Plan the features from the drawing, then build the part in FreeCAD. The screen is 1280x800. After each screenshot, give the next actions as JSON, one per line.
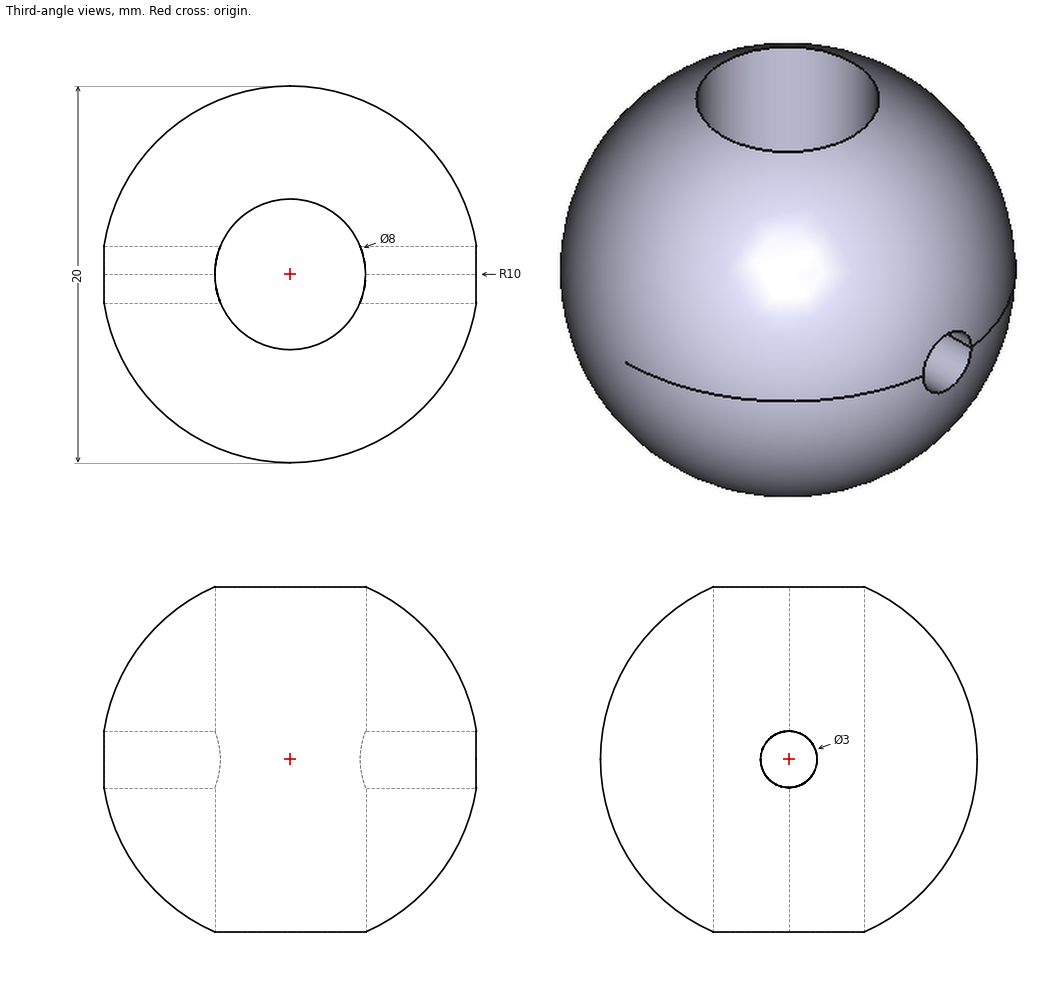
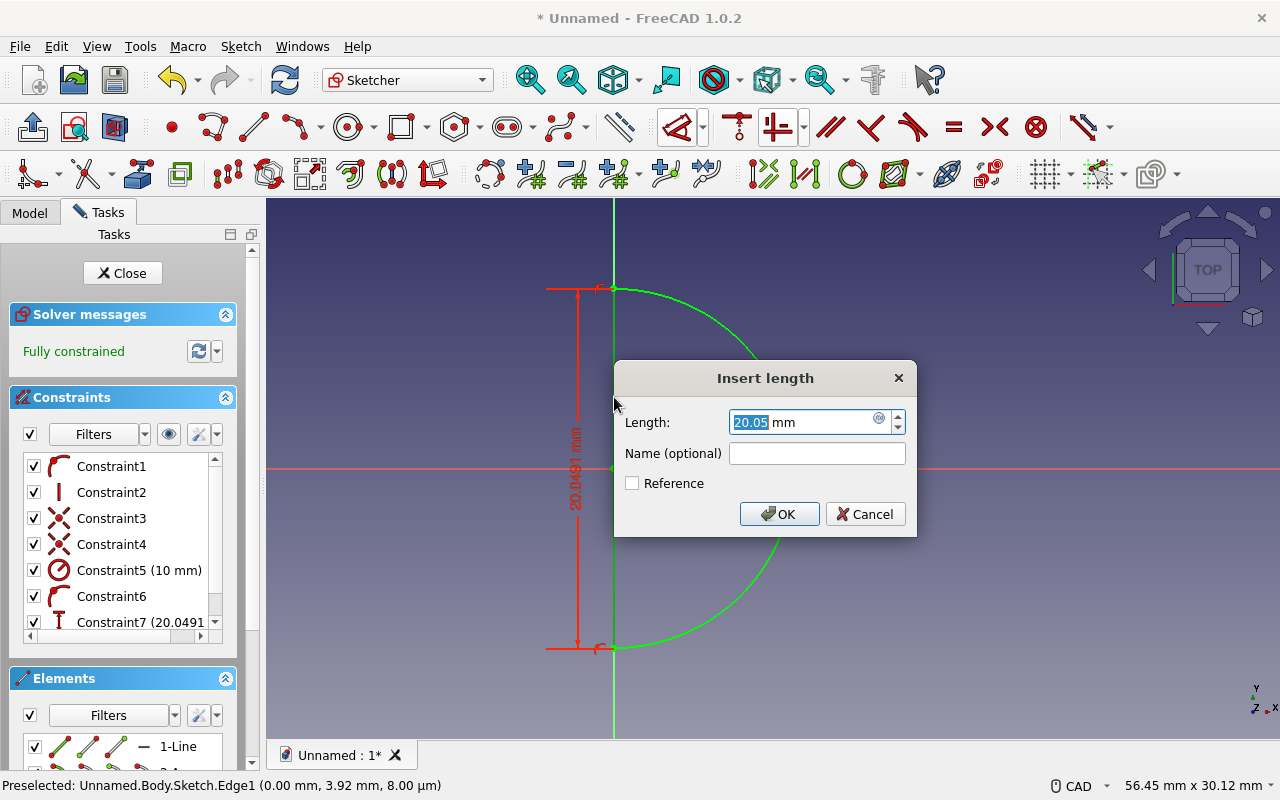
{"action": "type", "text": "20"}
{"action": "key", "text": "Return"}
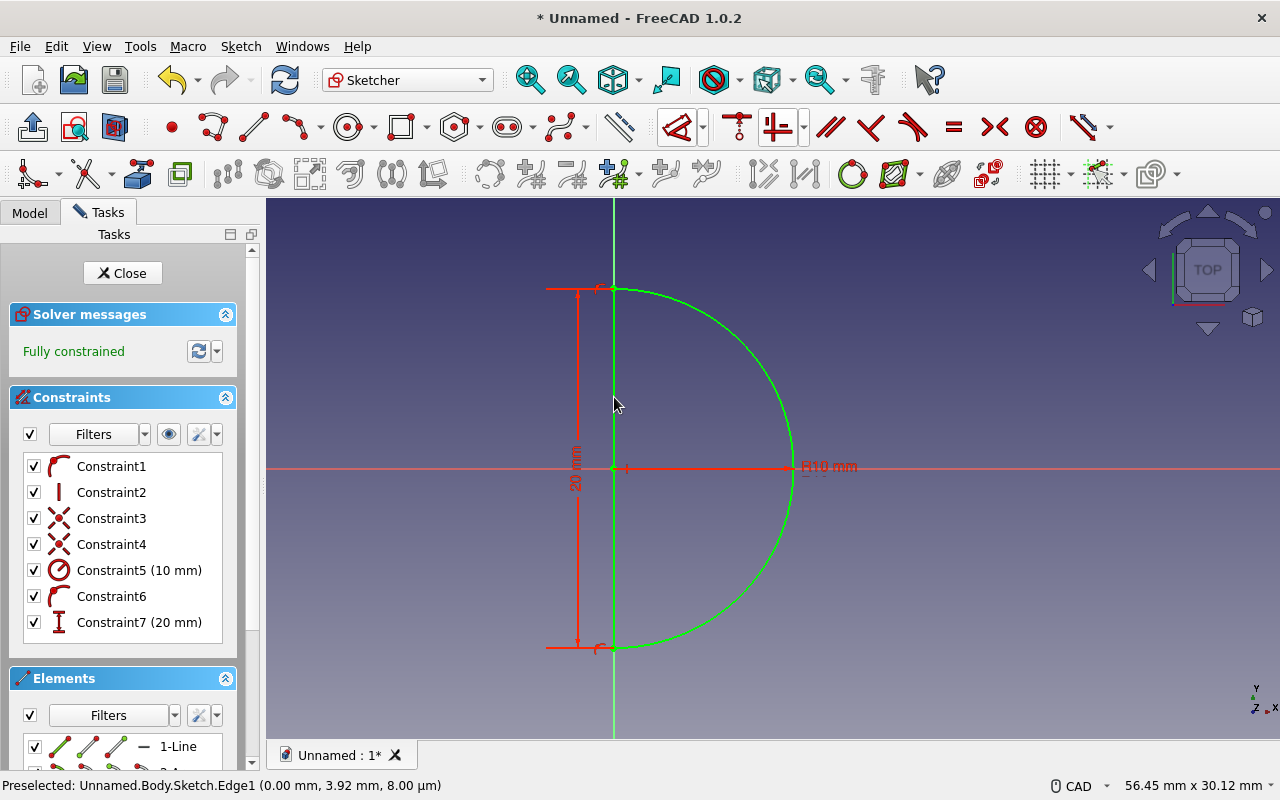
{"action": "left_click", "coordinate": [123, 273]}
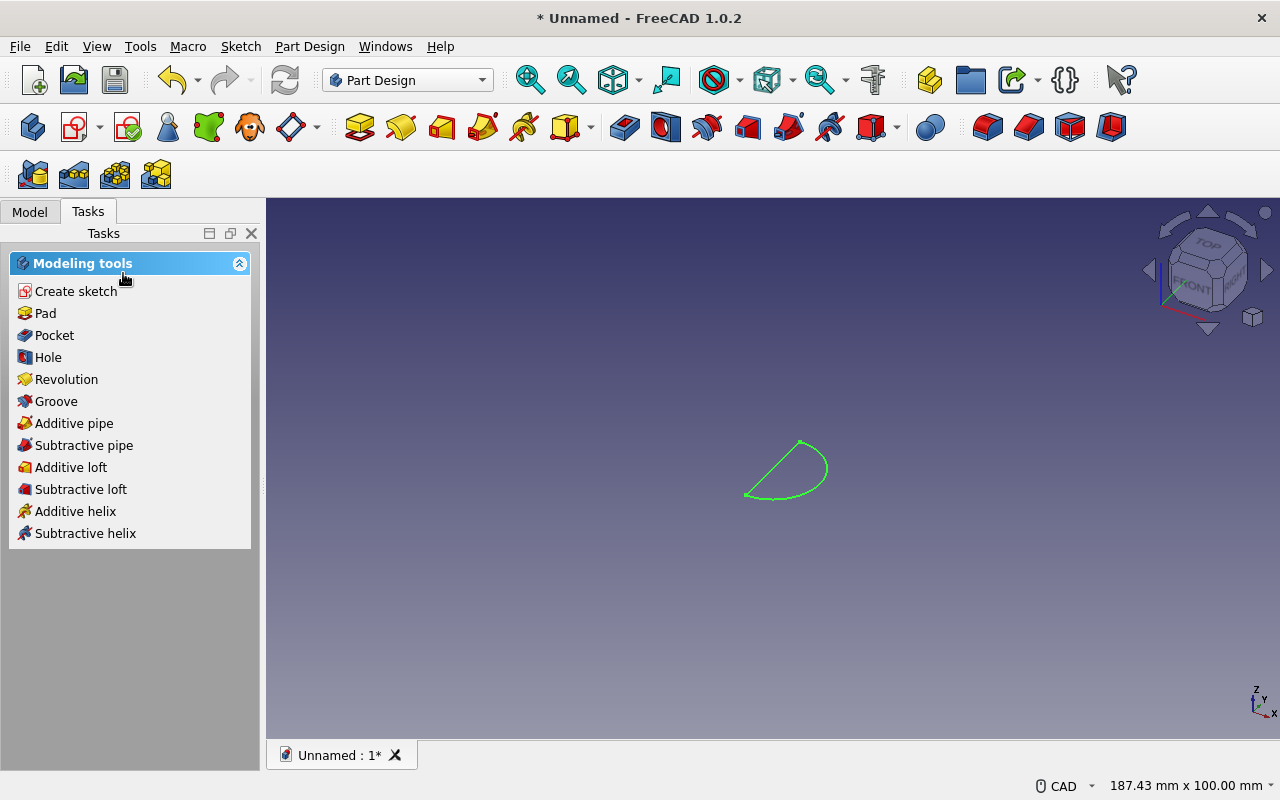
{"action": "left_click", "coordinate": [401, 128]}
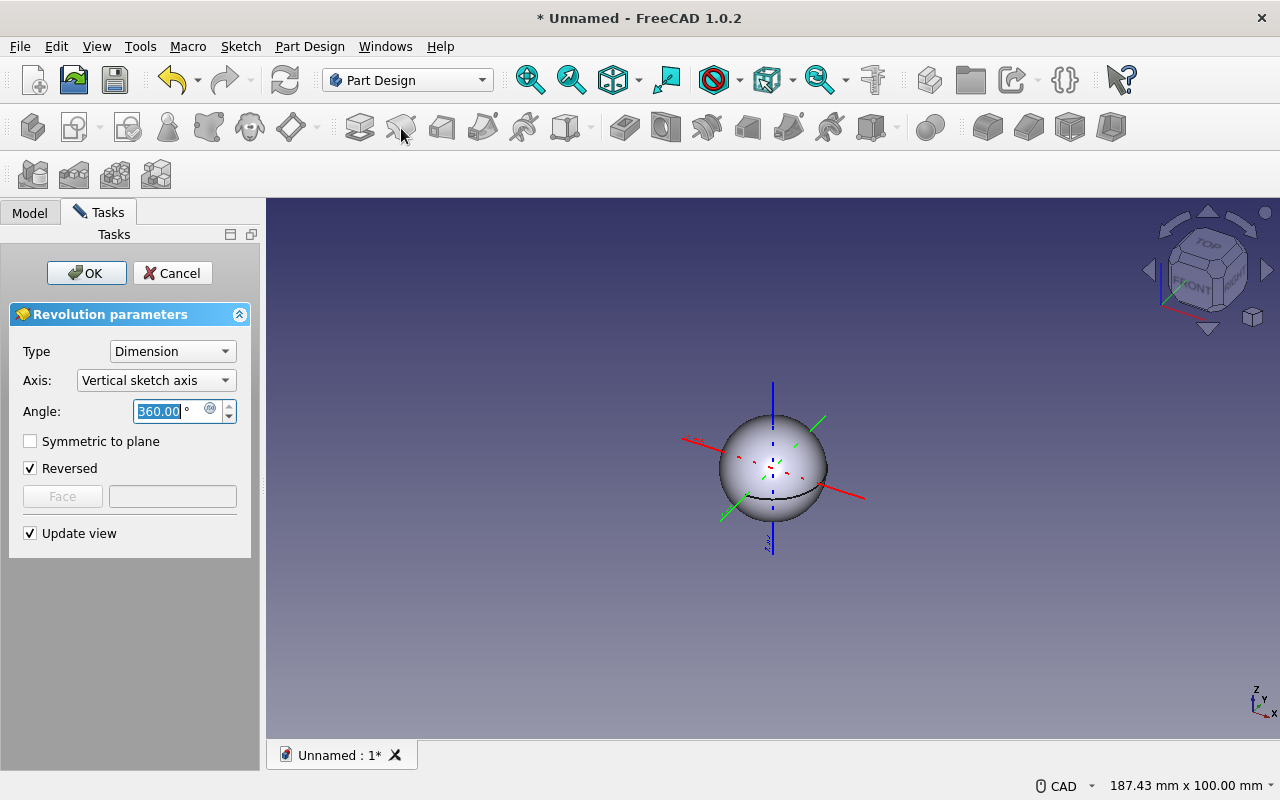
{"action": "left_click", "coordinate": [87, 273]}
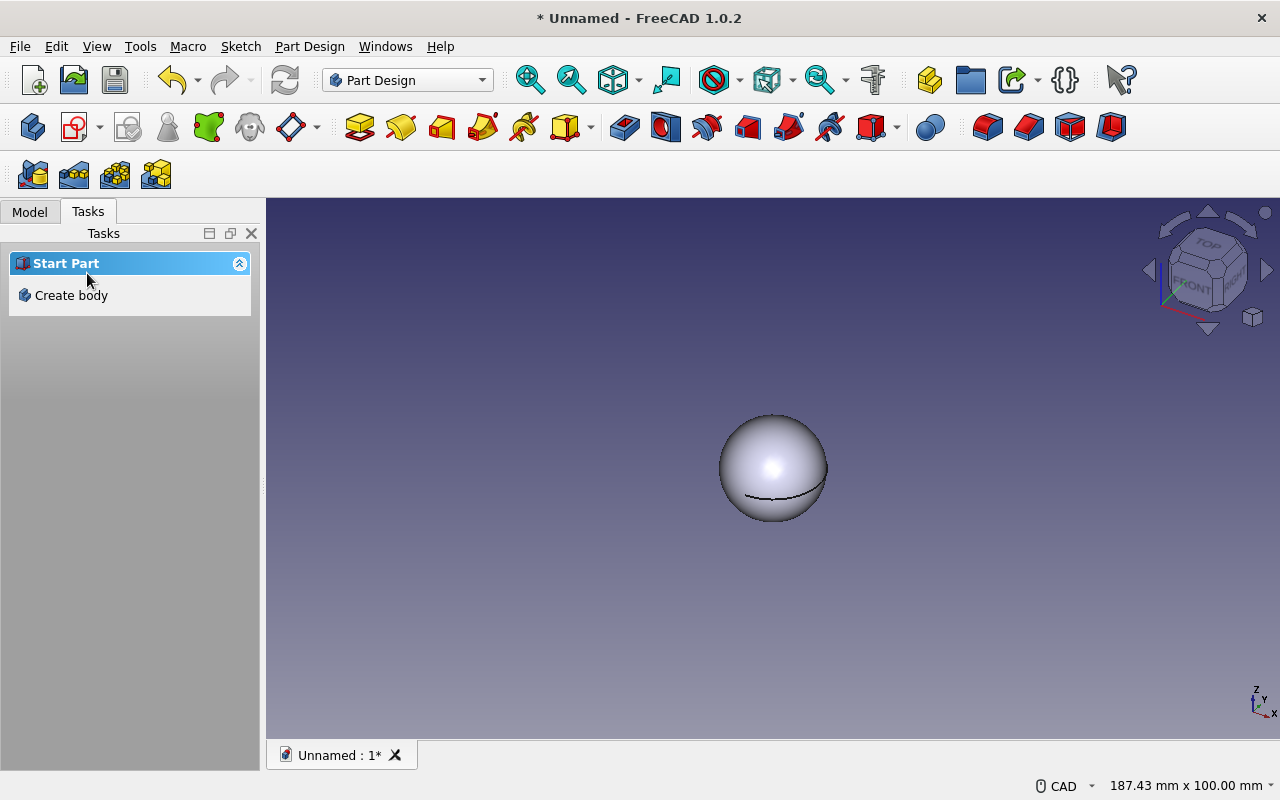
{"action": "left_click", "coordinate": [531, 80]}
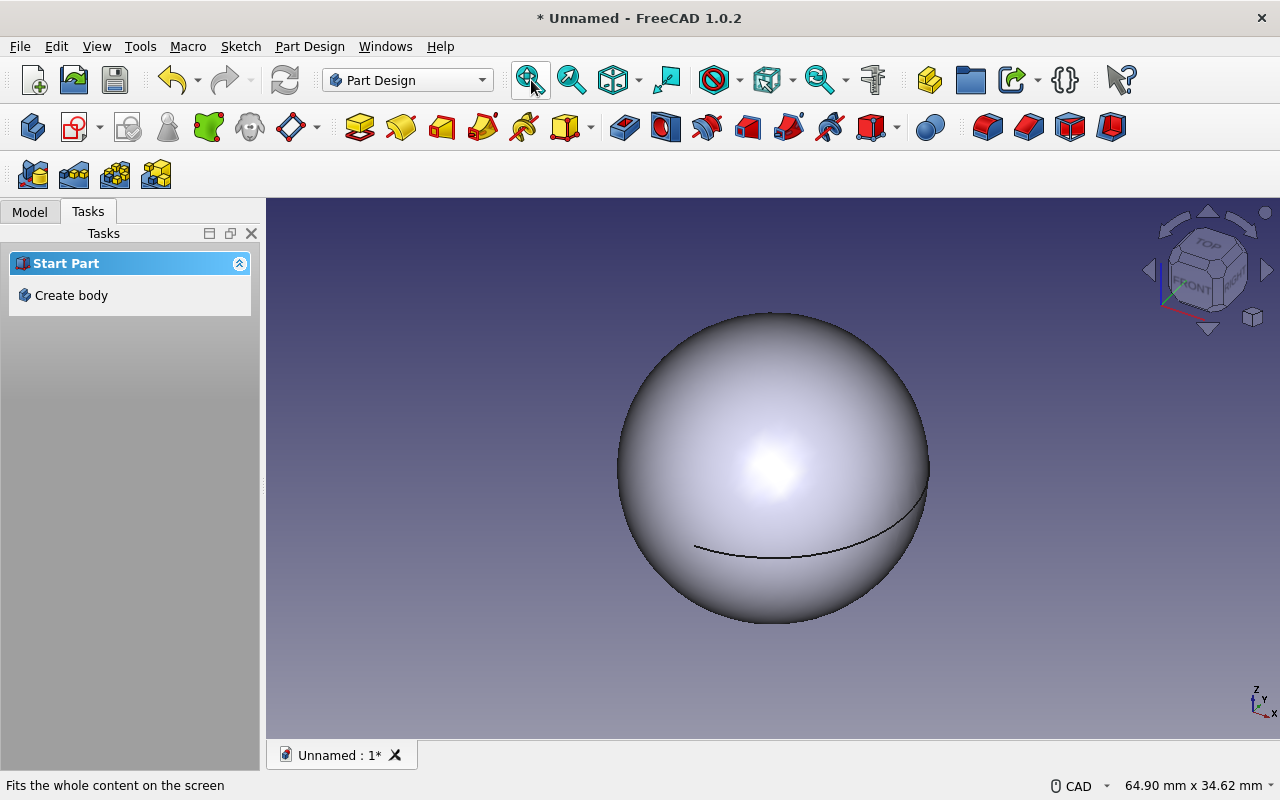
{"action": "left_click", "coordinate": [74, 128]}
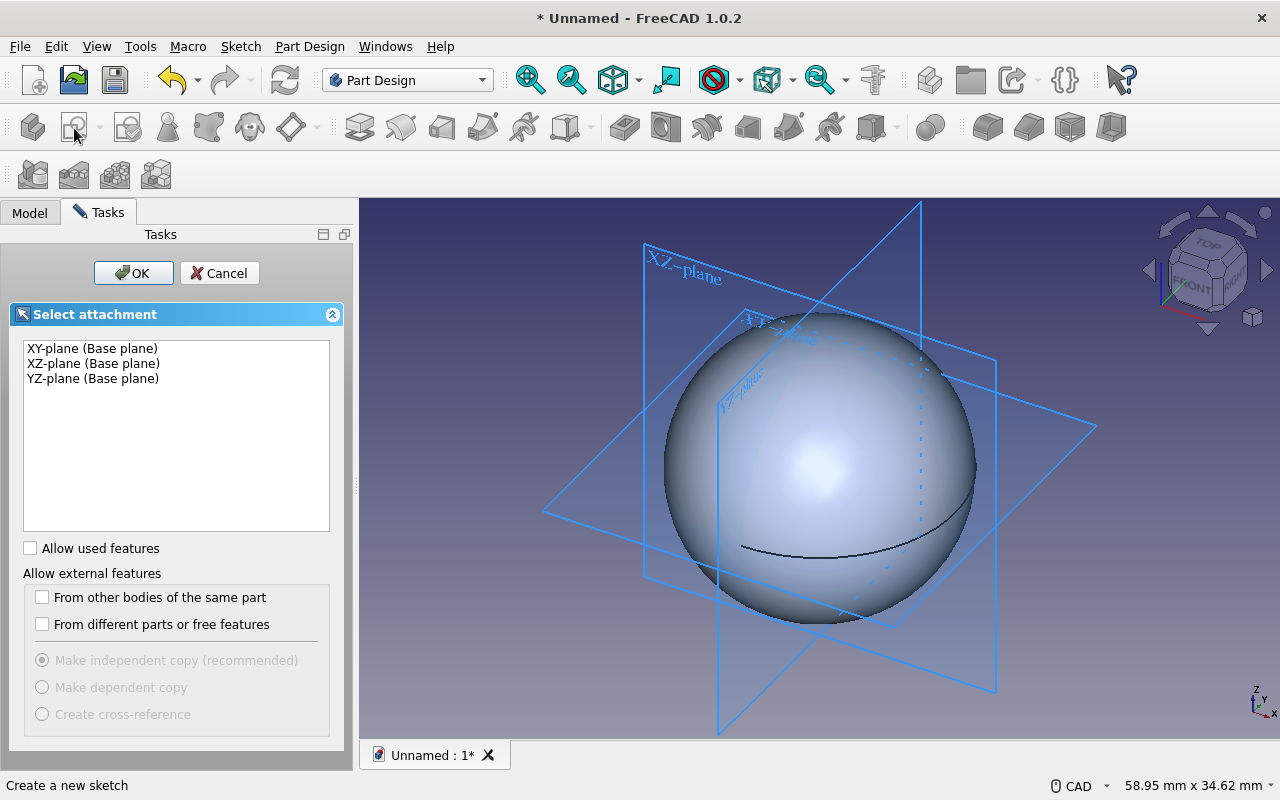
{"action": "left_click", "coordinate": [84, 348]}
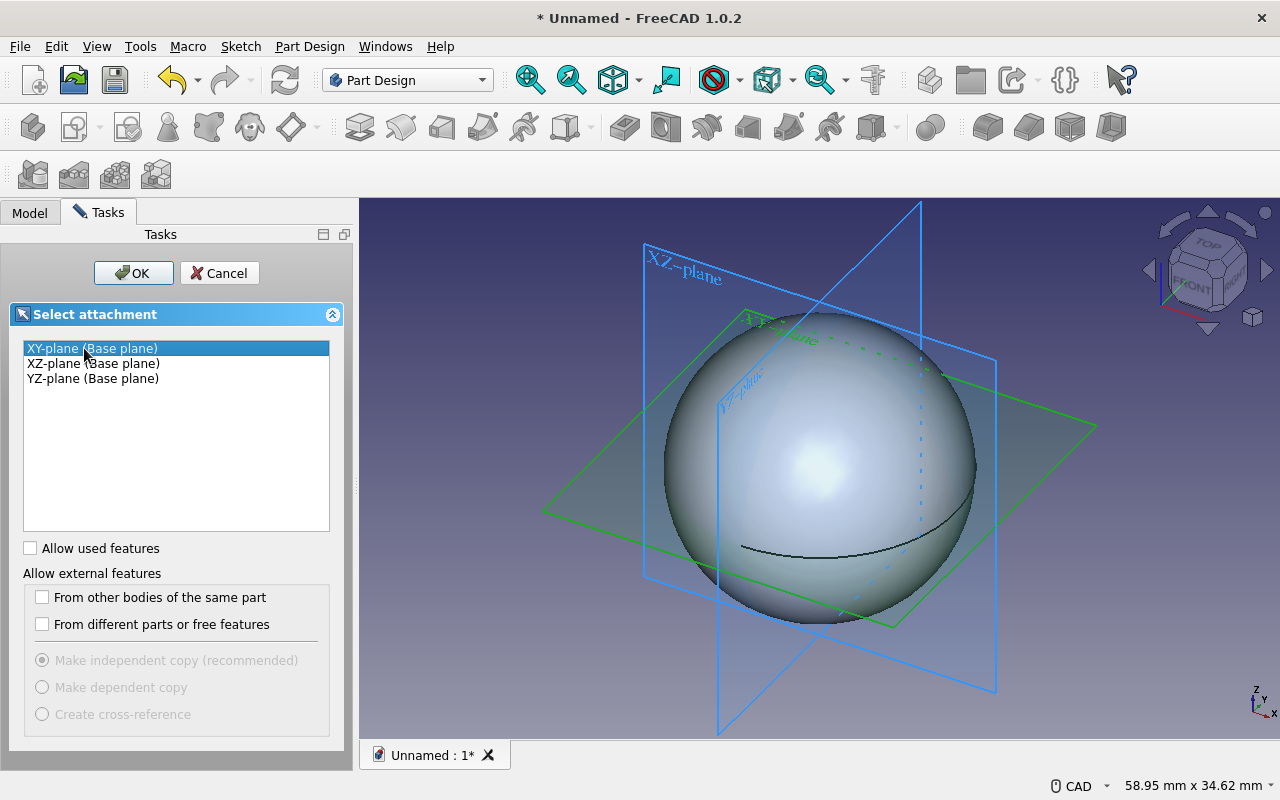
{"action": "left_click", "coordinate": [134, 273]}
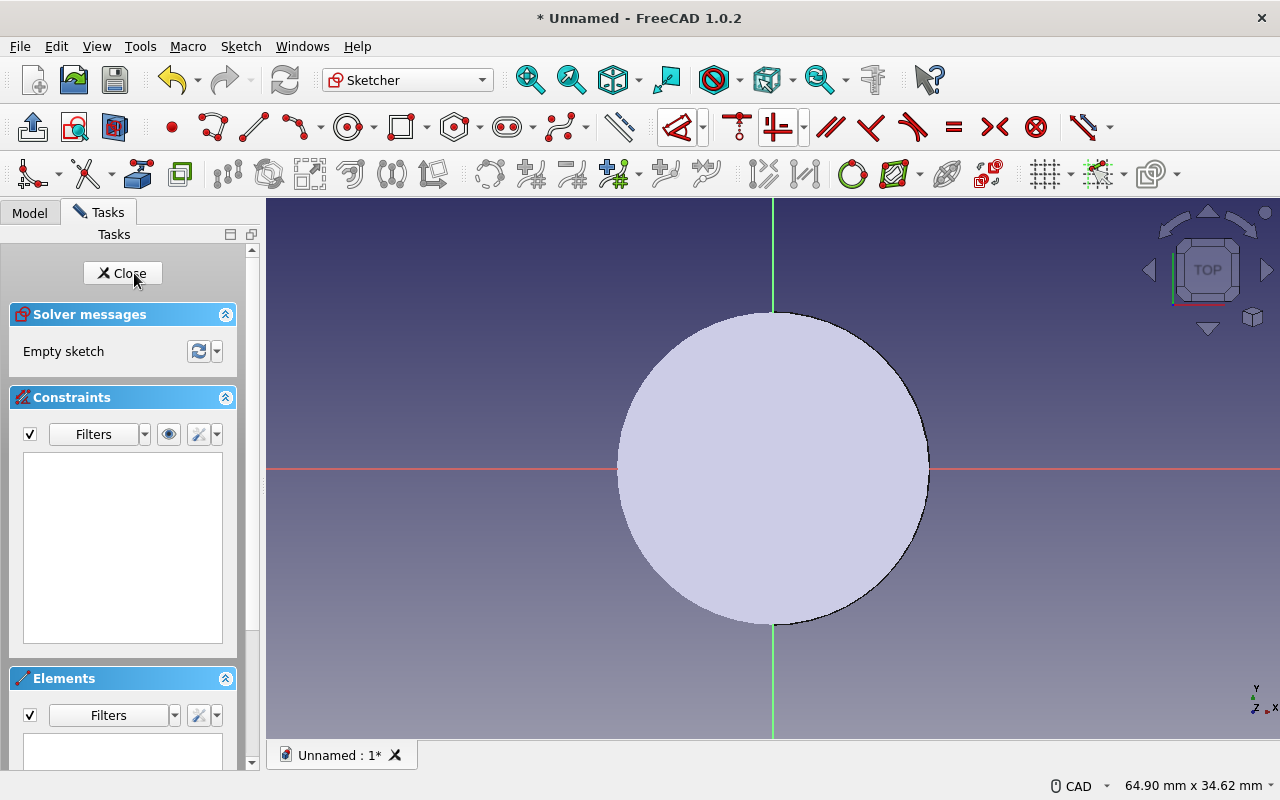
{"action": "left_click", "coordinate": [115, 128]}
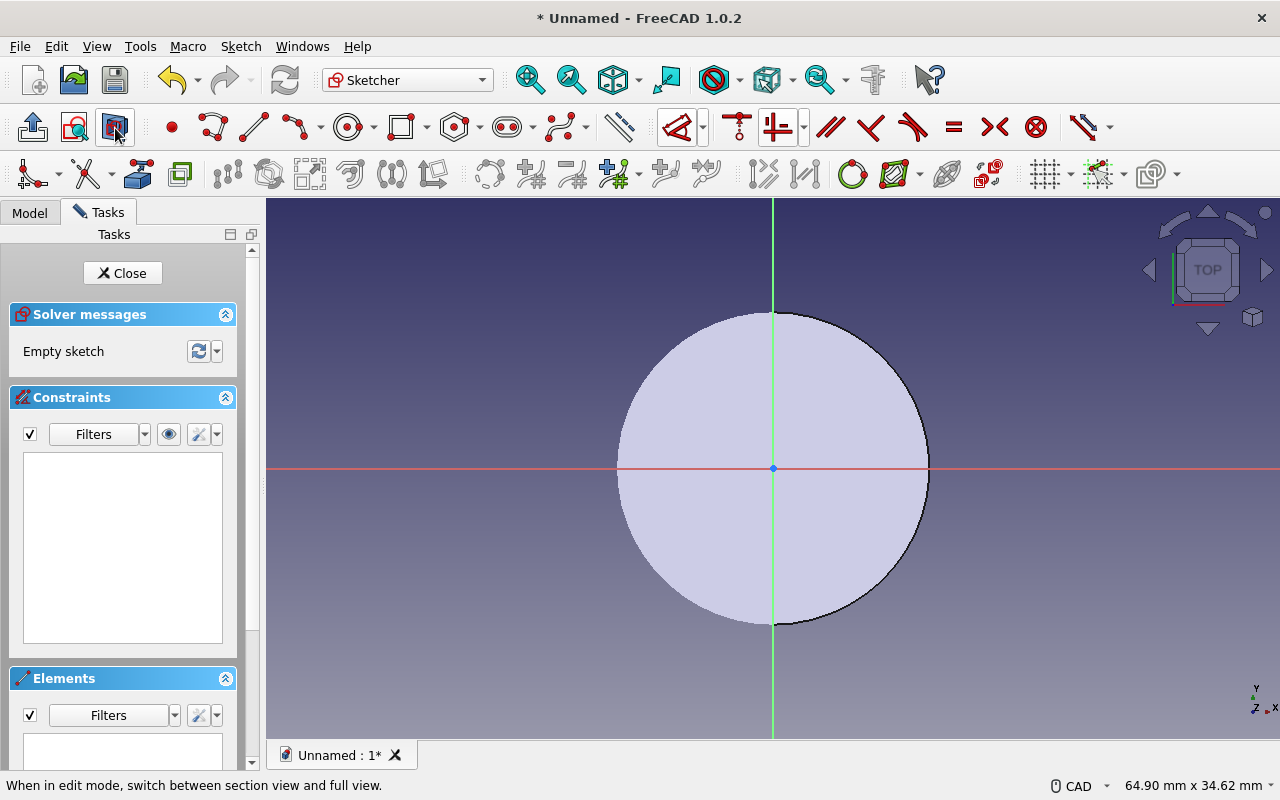
{"action": "scroll", "coordinate": [813, 468], "scroll_direction": "up", "scroll_amount": 5}